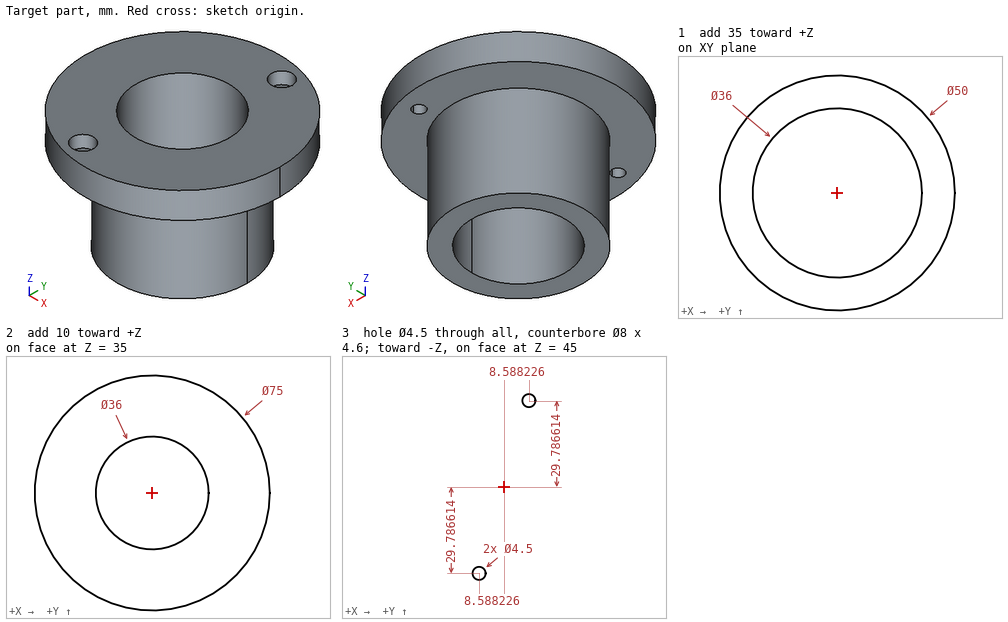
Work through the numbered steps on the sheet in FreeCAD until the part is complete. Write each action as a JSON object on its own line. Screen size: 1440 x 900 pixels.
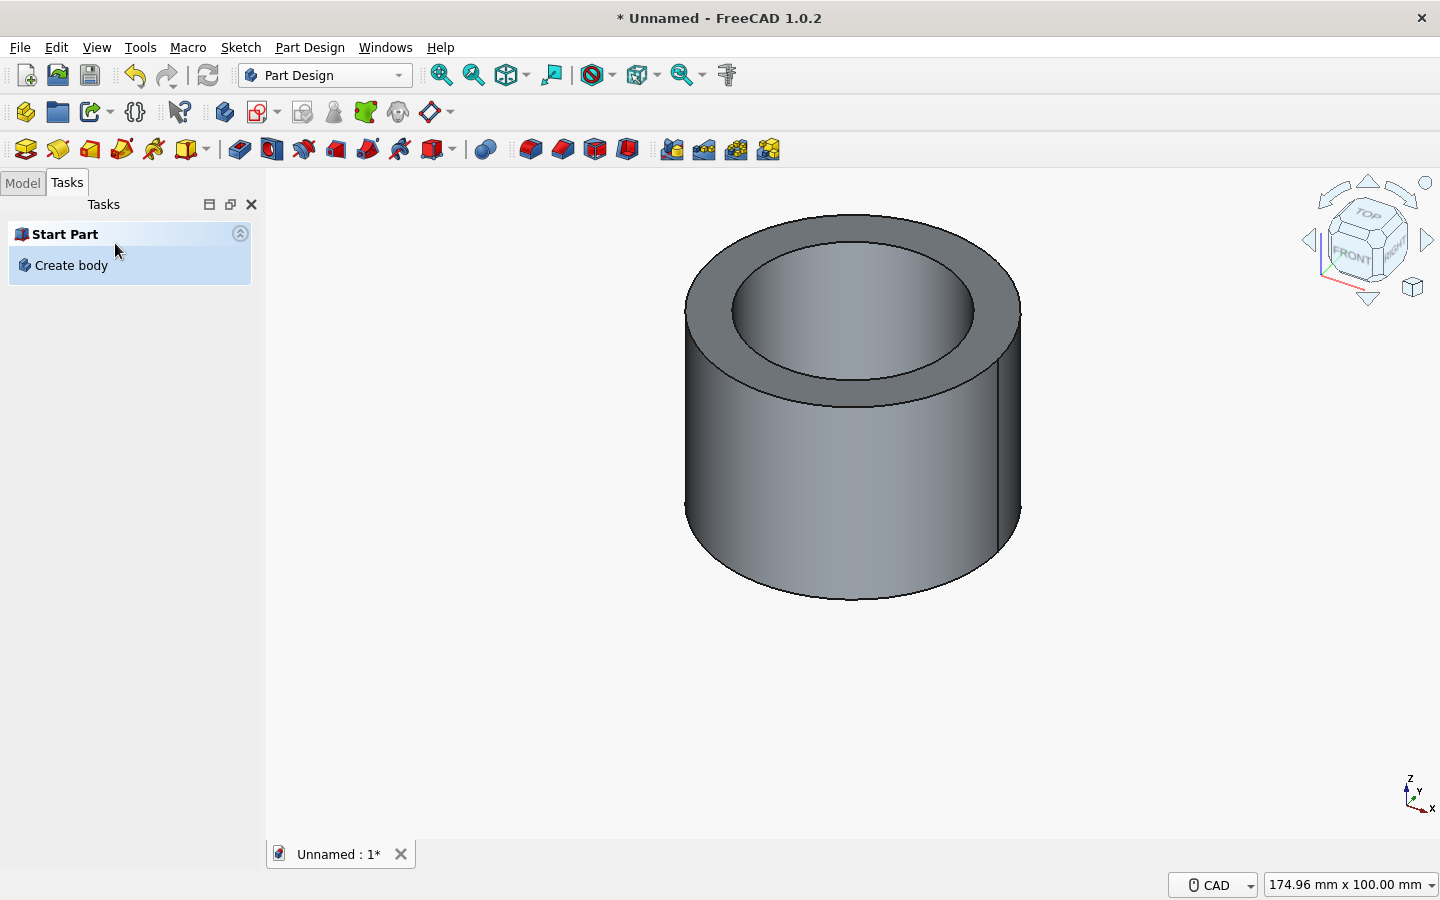
{"action": "left_click", "coordinate": [978, 351]}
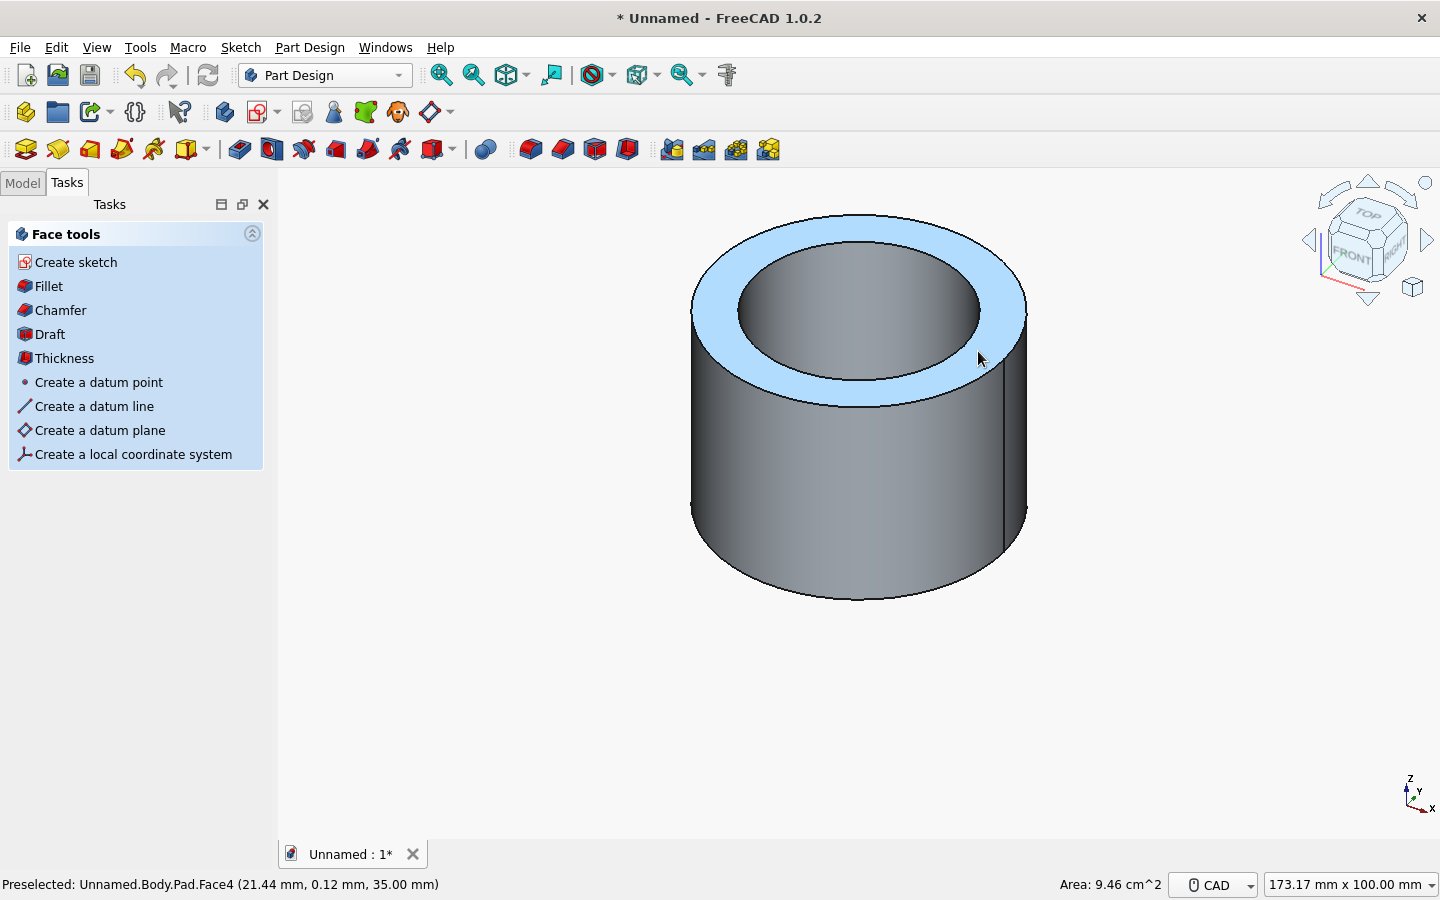
{"action": "left_click", "coordinate": [258, 112]}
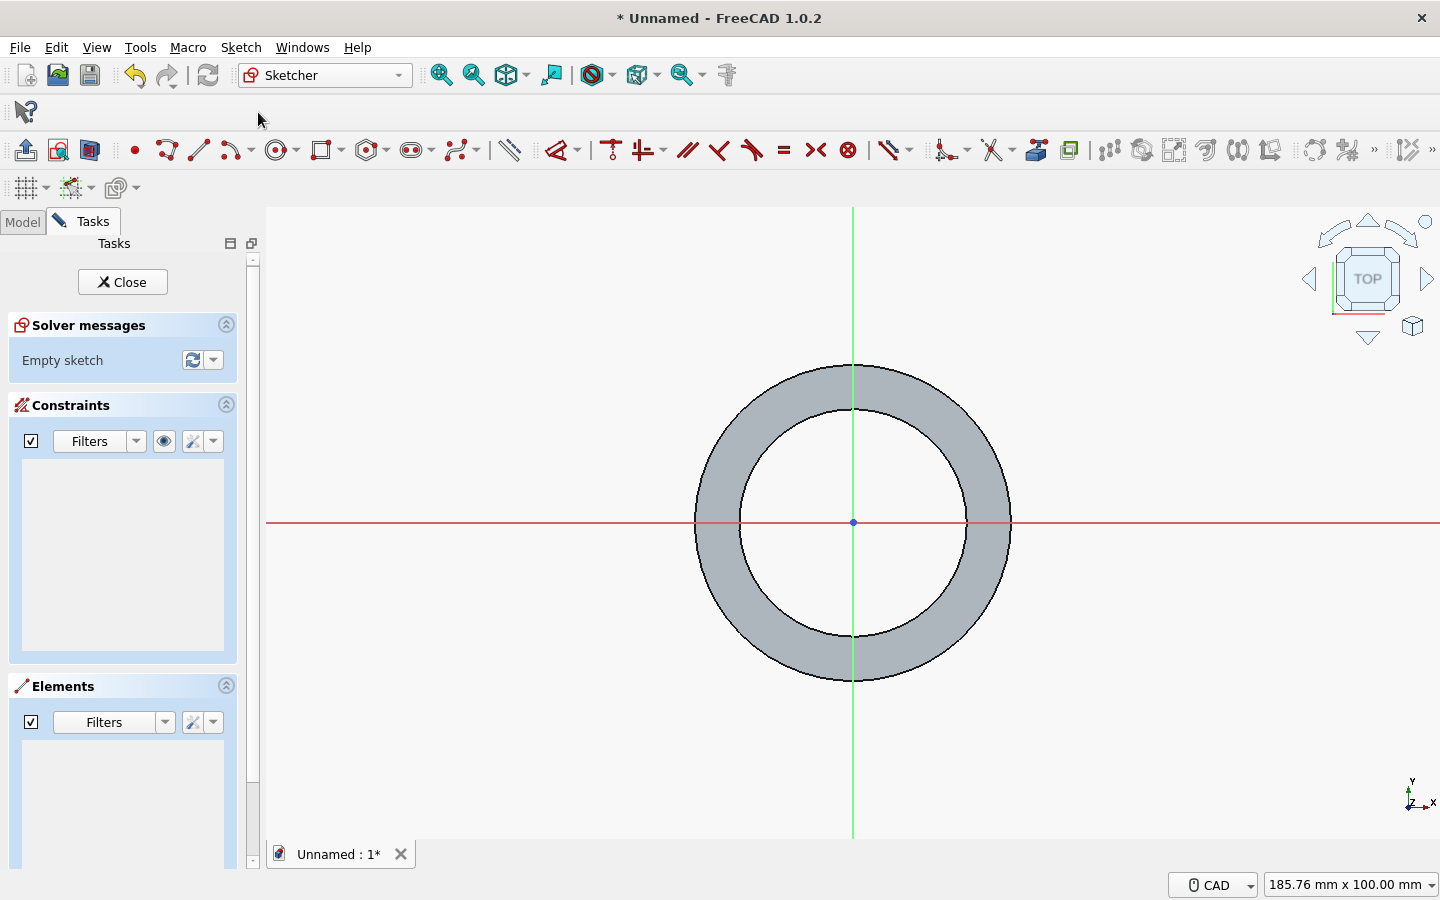
{"action": "key", "text": "g c"}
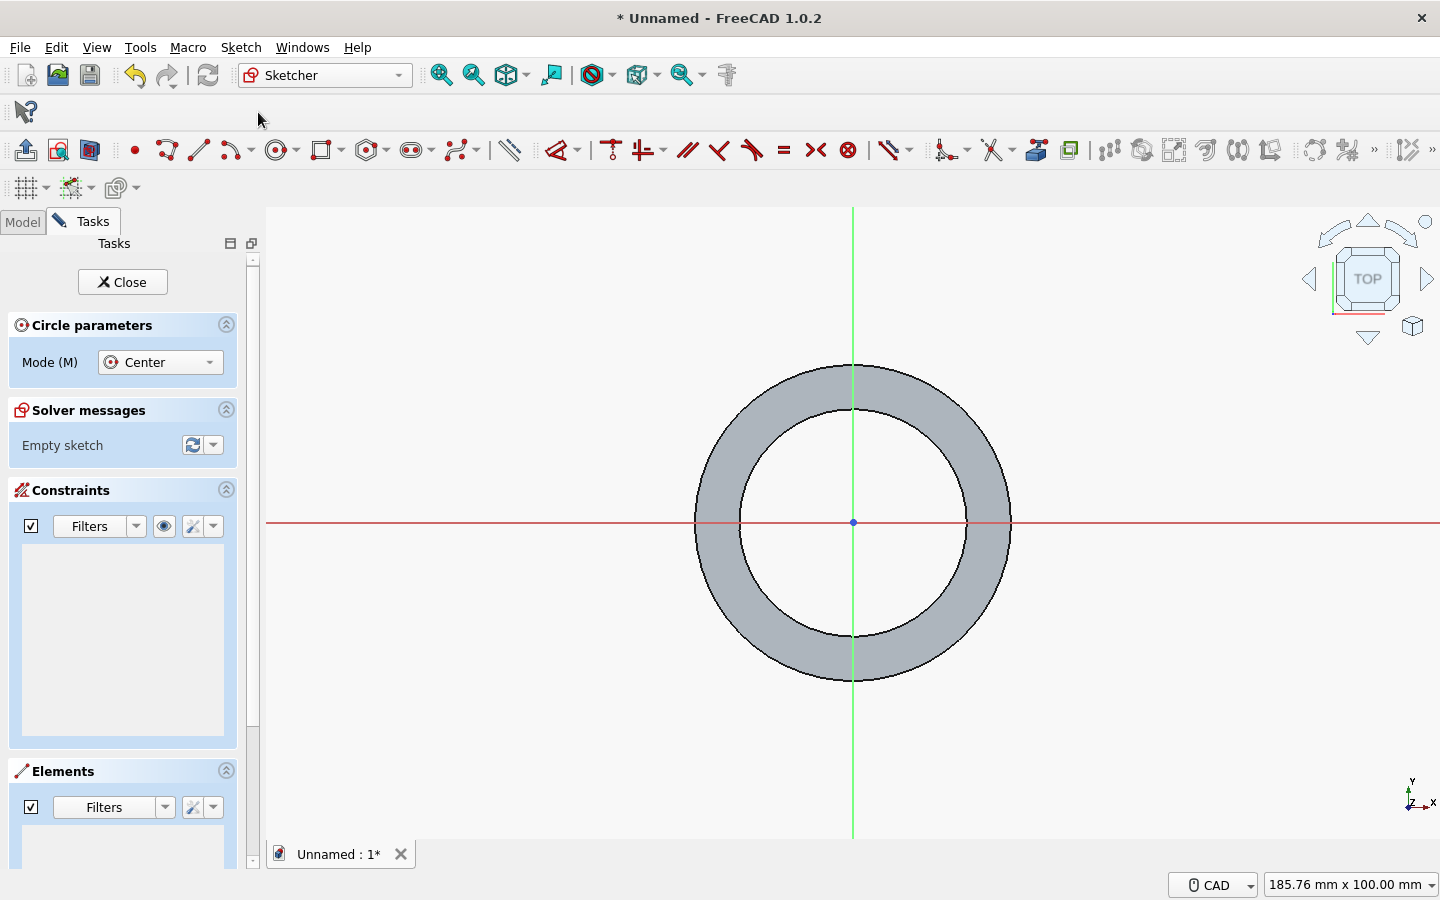
{"action": "left_click", "coordinate": [853, 523]}
{"action": "left_click", "coordinate": [1021, 355]}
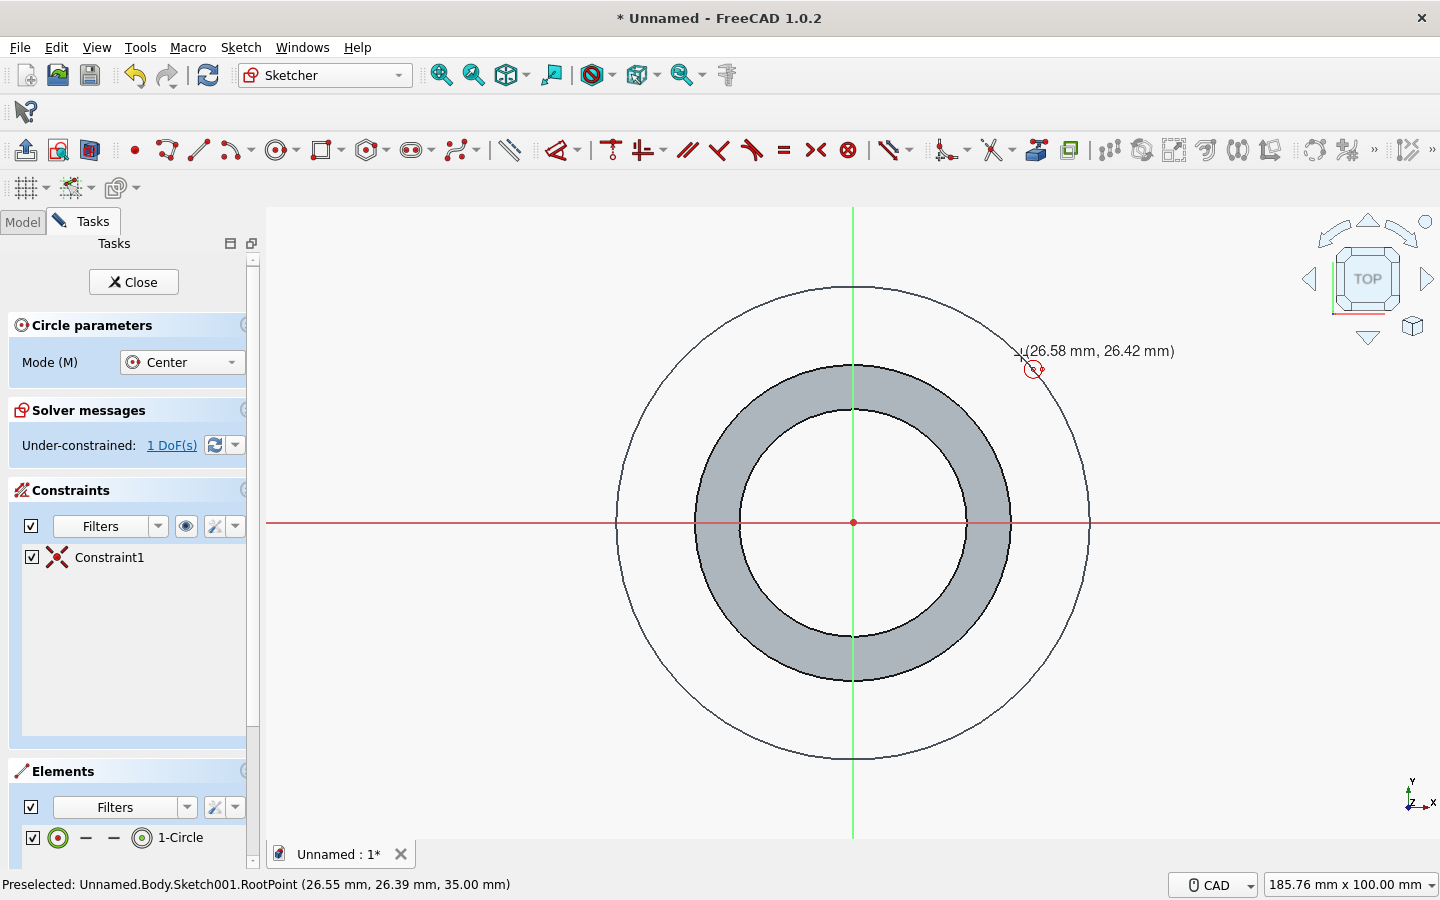
{"action": "left_click", "coordinate": [853, 523]}
{"action": "left_click", "coordinate": [933, 443]}
{"action": "key", "text": "Escape"}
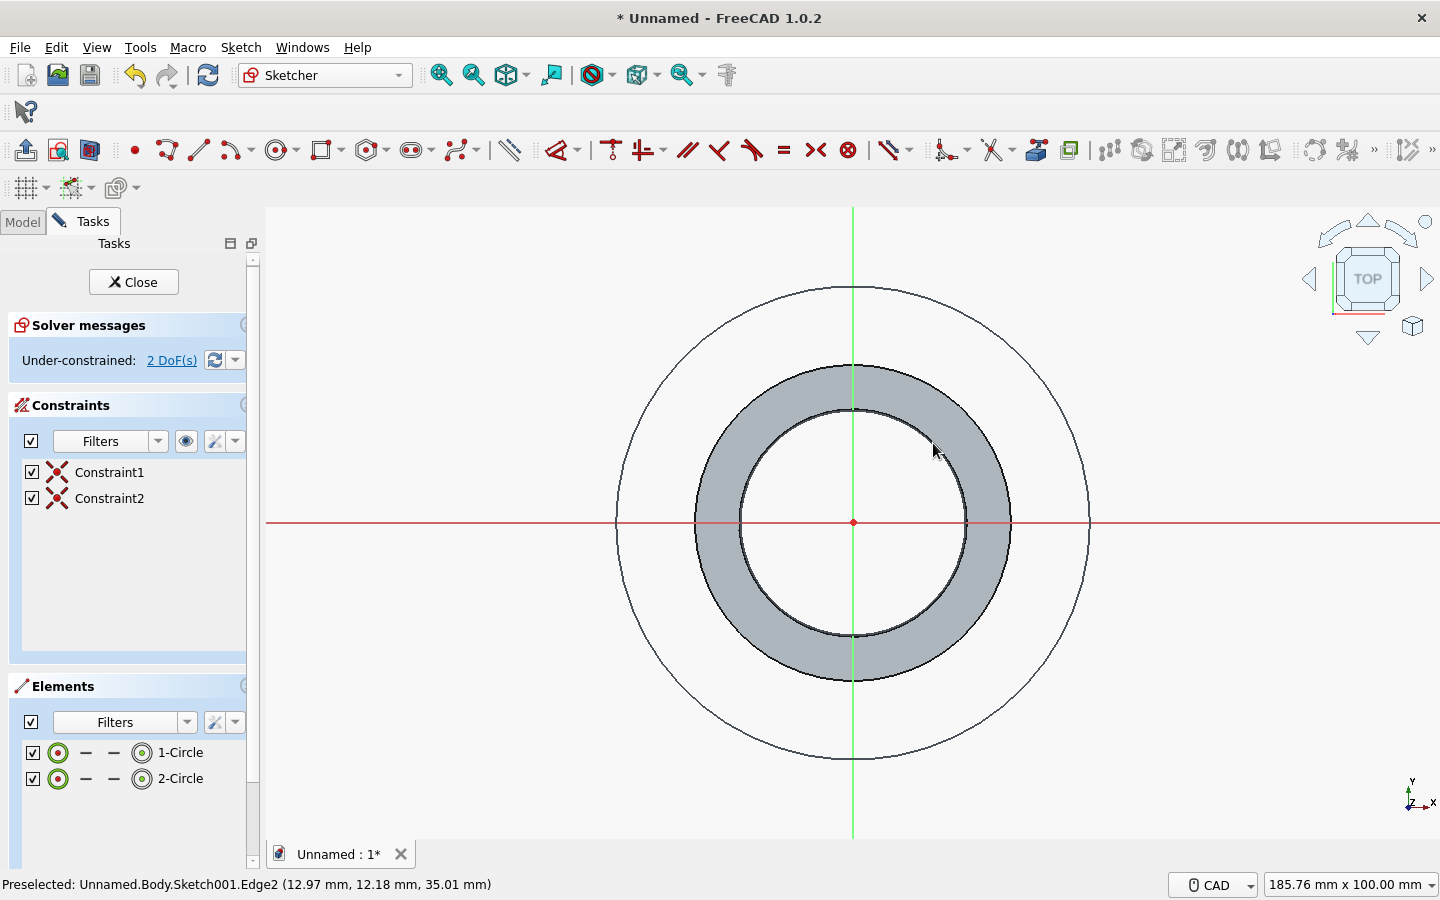
{"action": "key", "text": "d"}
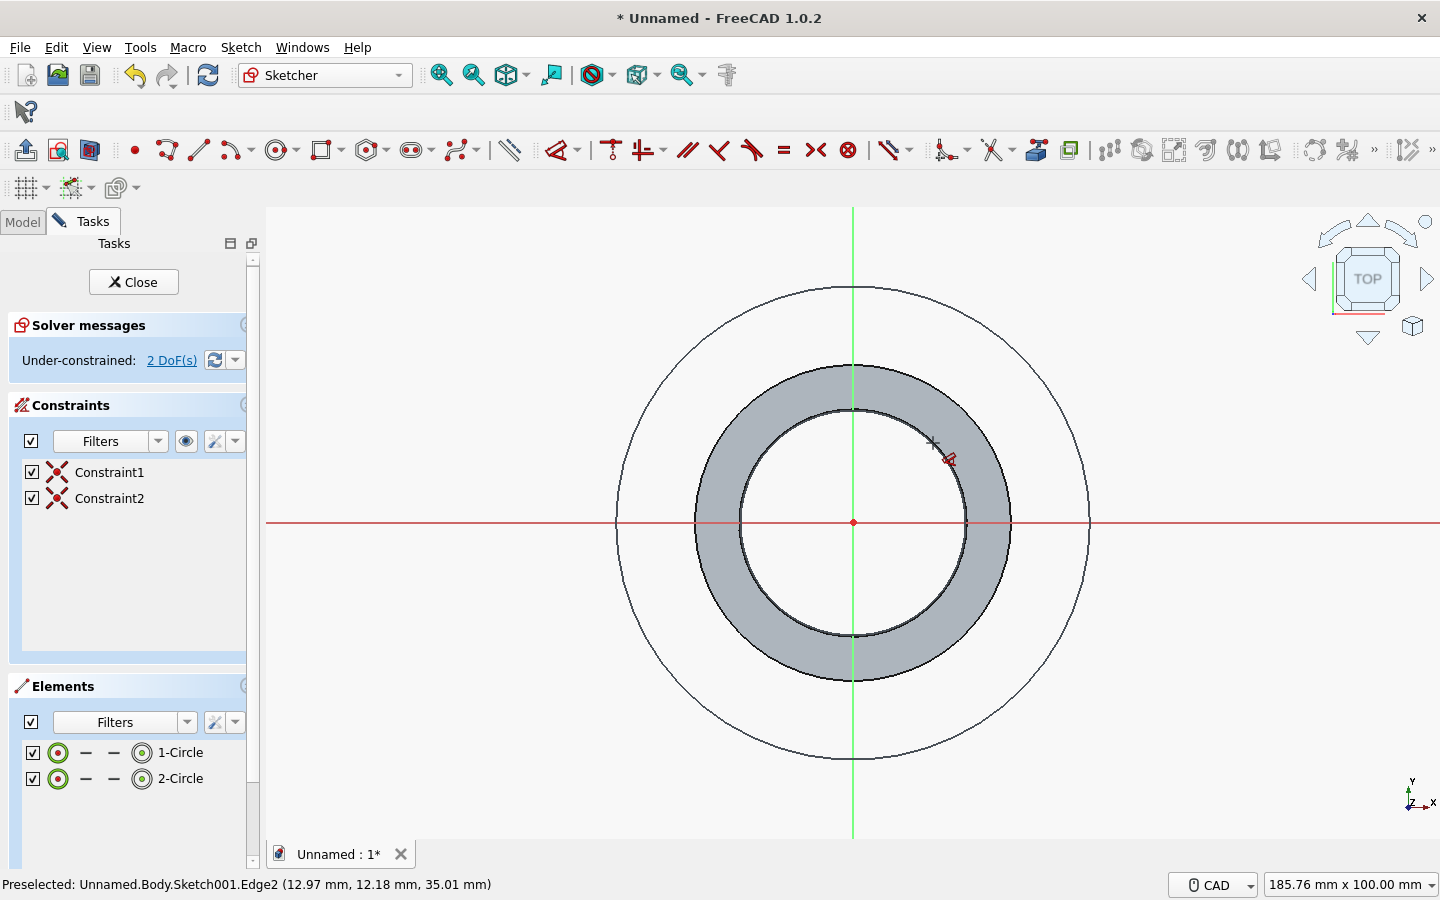
{"action": "left_click", "coordinate": [1020, 355]}
{"action": "left_click", "coordinate": [1043, 332]}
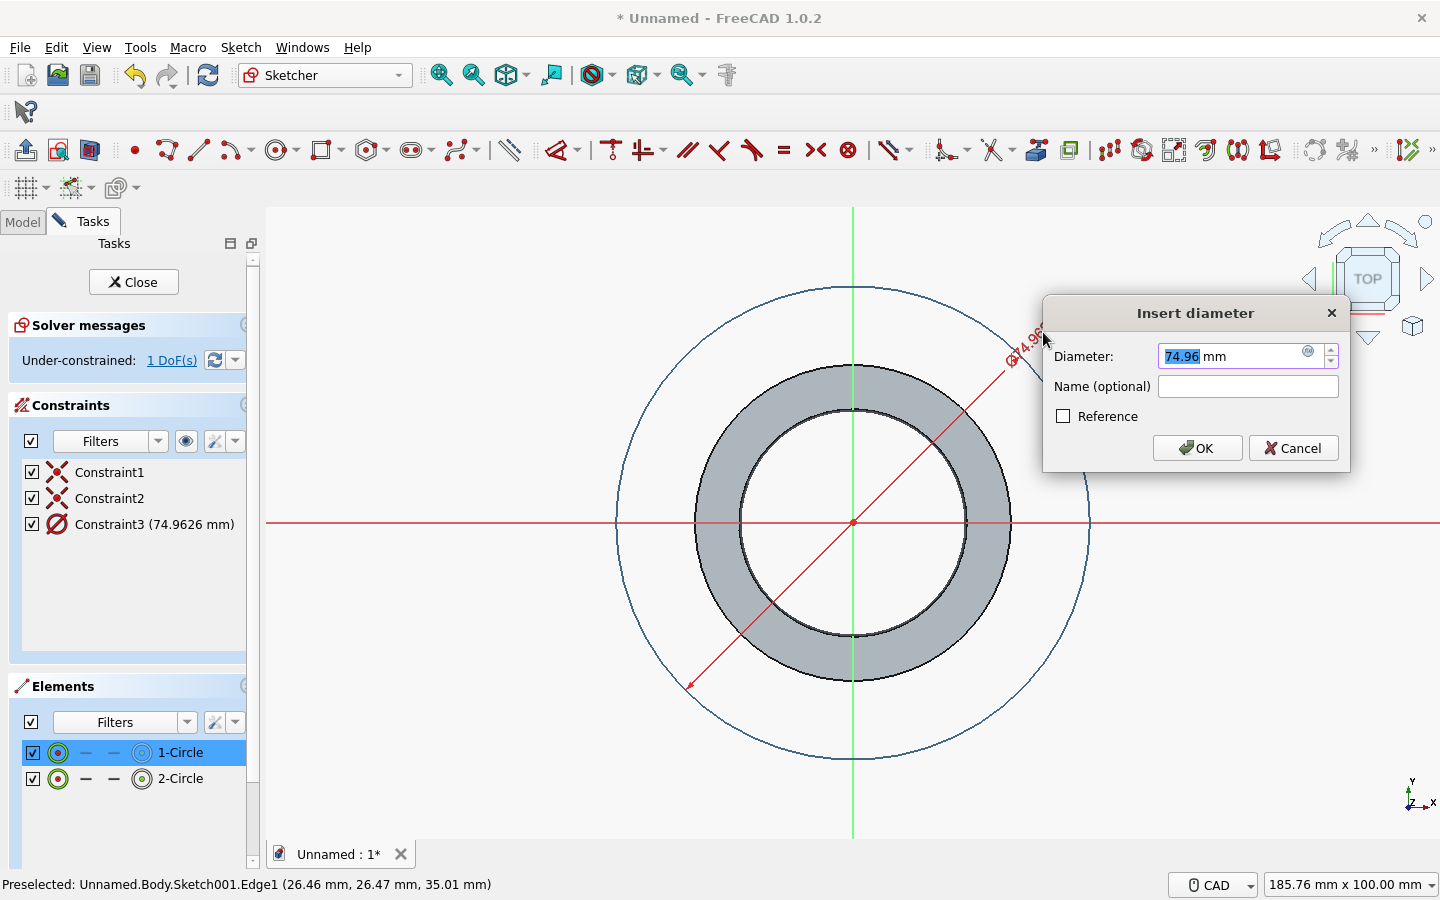
{"action": "type", "text": "75"}
{"action": "key", "text": "Return"}